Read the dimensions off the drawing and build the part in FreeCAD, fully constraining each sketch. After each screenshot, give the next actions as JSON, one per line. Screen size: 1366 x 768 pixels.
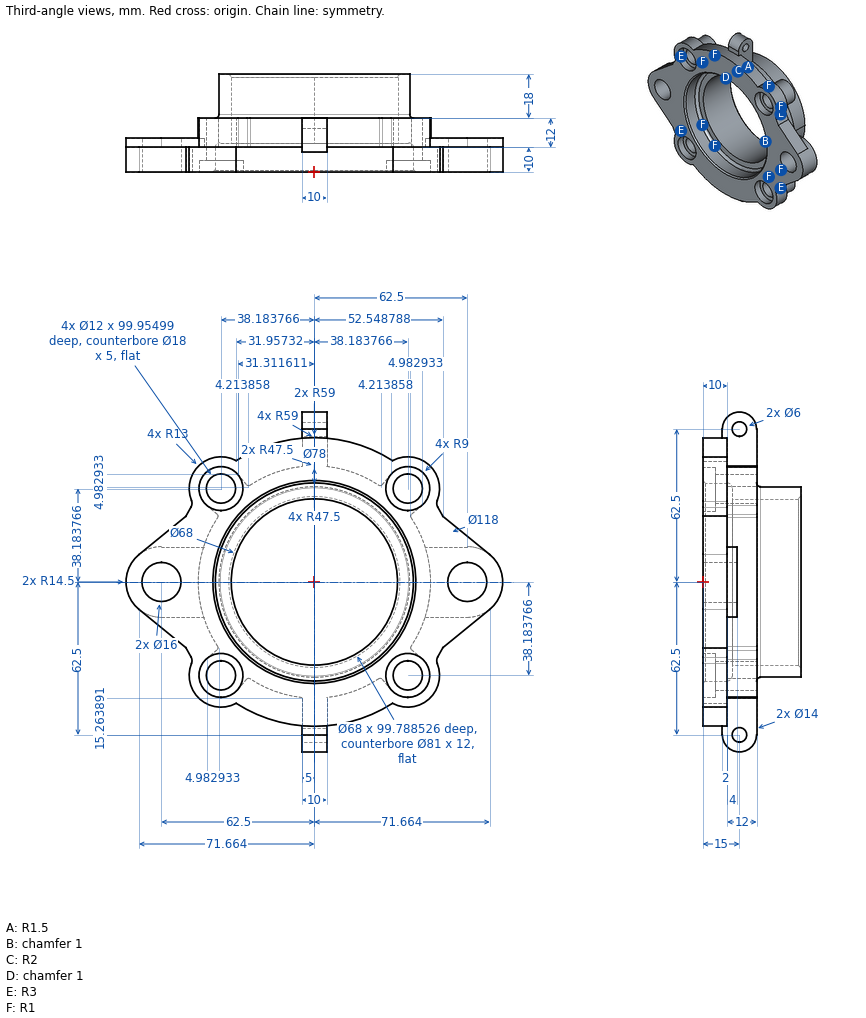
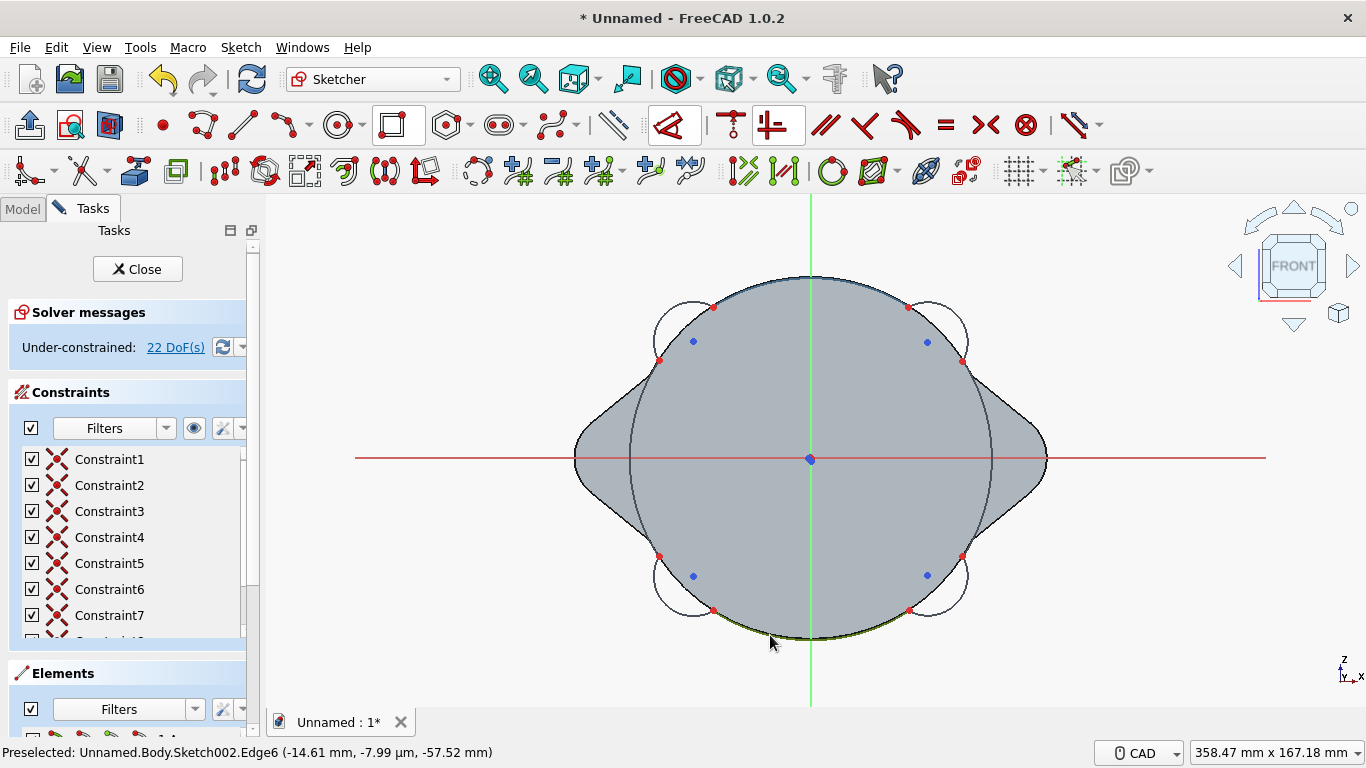
{"action": "left_click", "coordinate": [732, 126]}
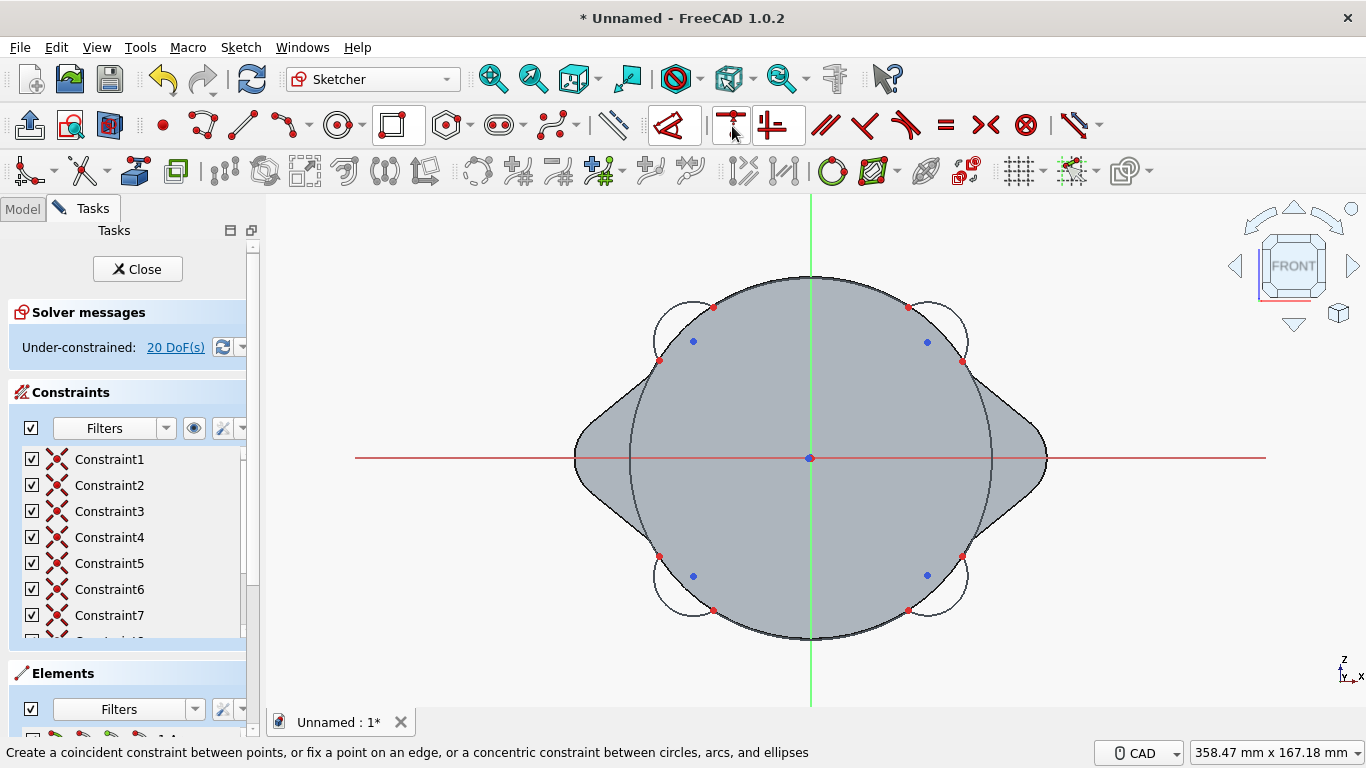
{"action": "left_click", "coordinate": [852, 283]}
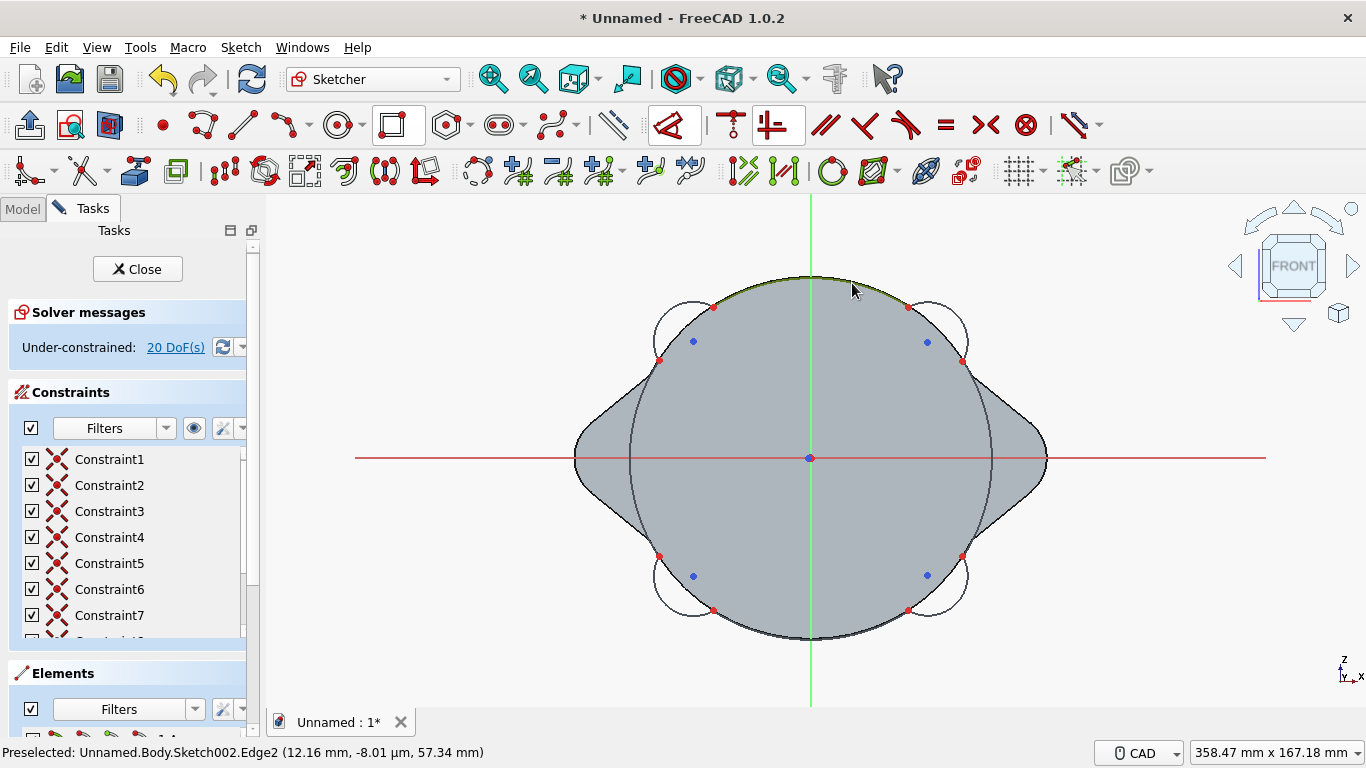
{"action": "left_click", "coordinate": [635, 418]}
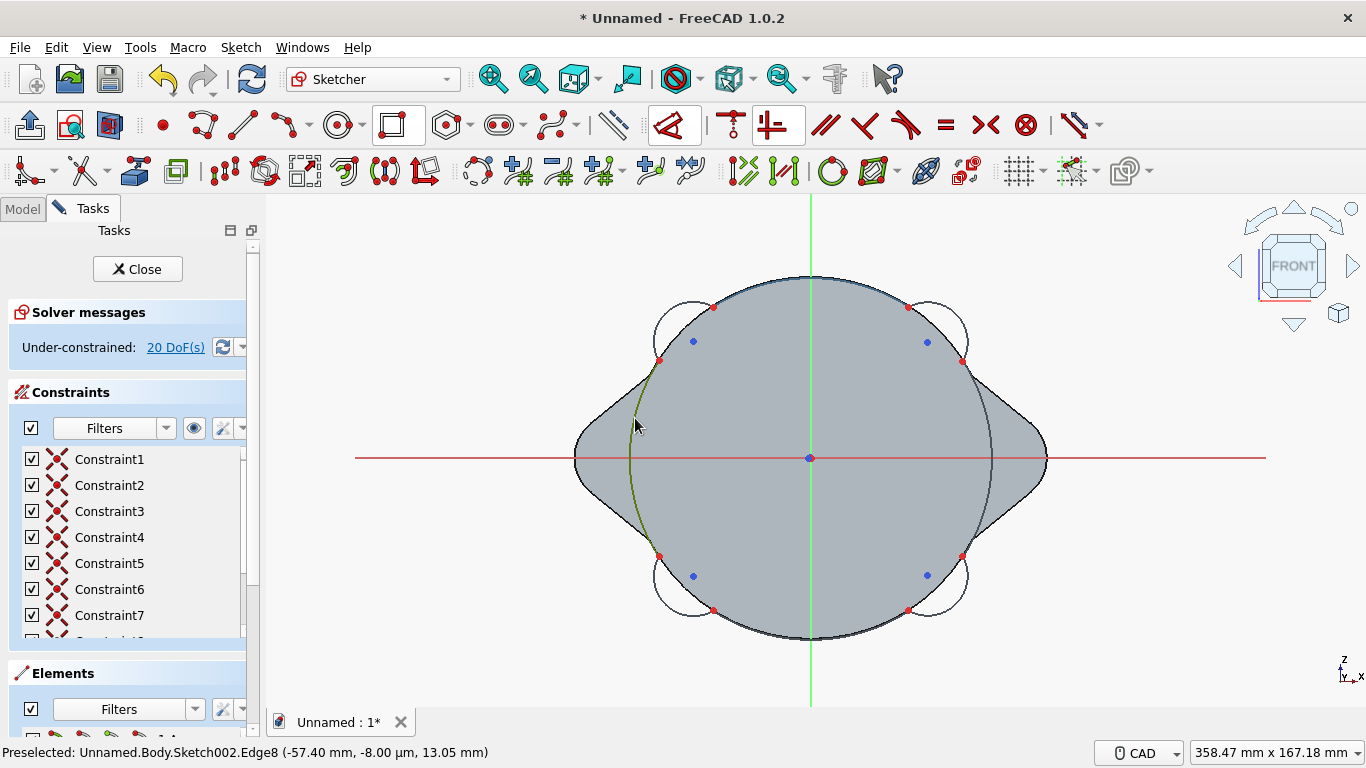
{"action": "left_click", "coordinate": [732, 126]}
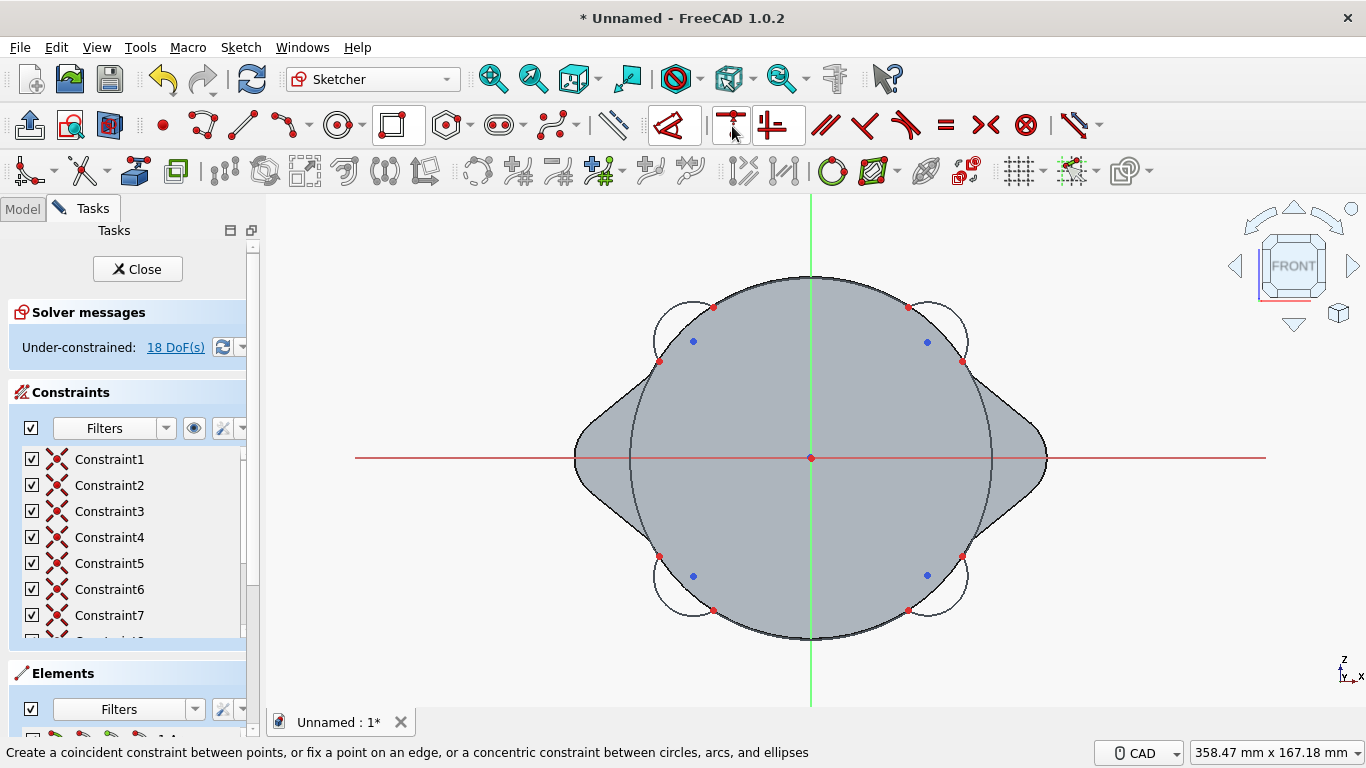
{"action": "left_click_drag", "start_coordinate": [801, 448], "coordinate": [821, 469]}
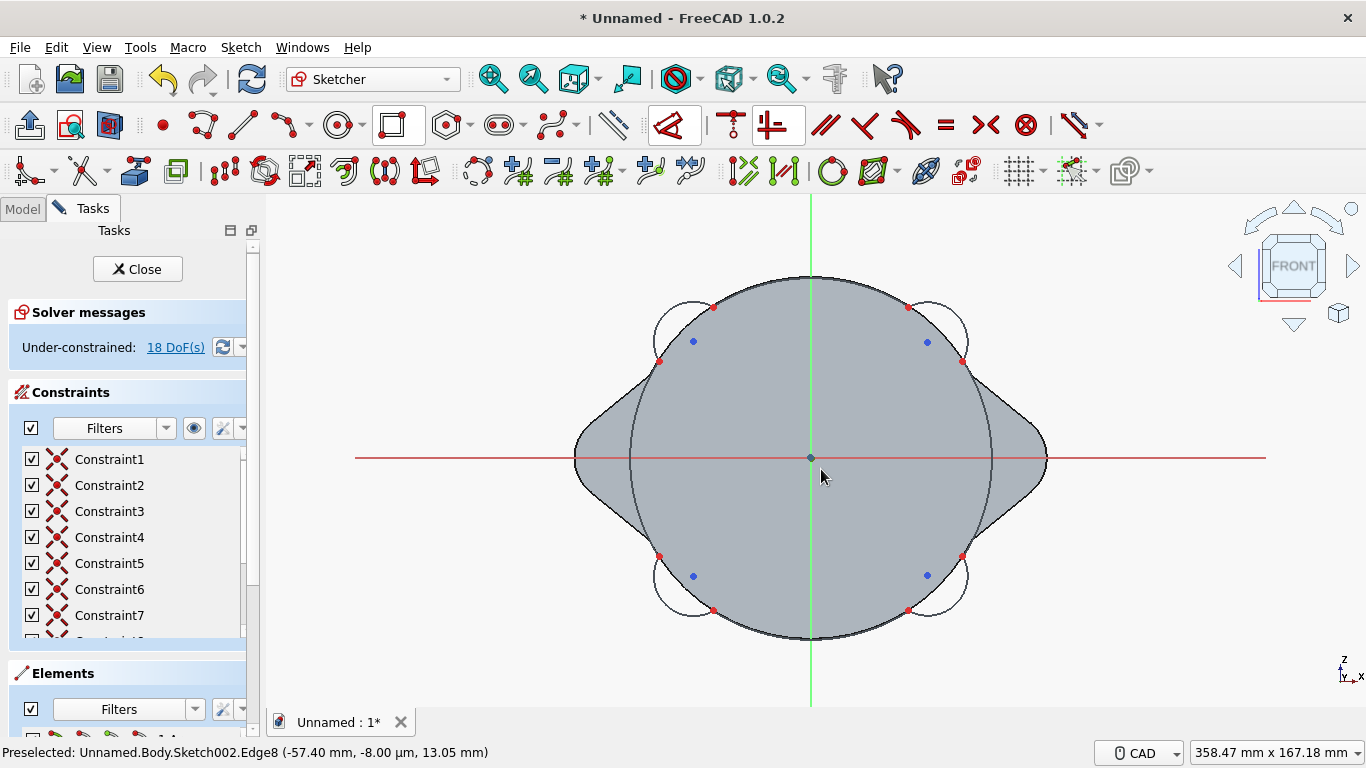
{"action": "left_click", "coordinate": [732, 126]}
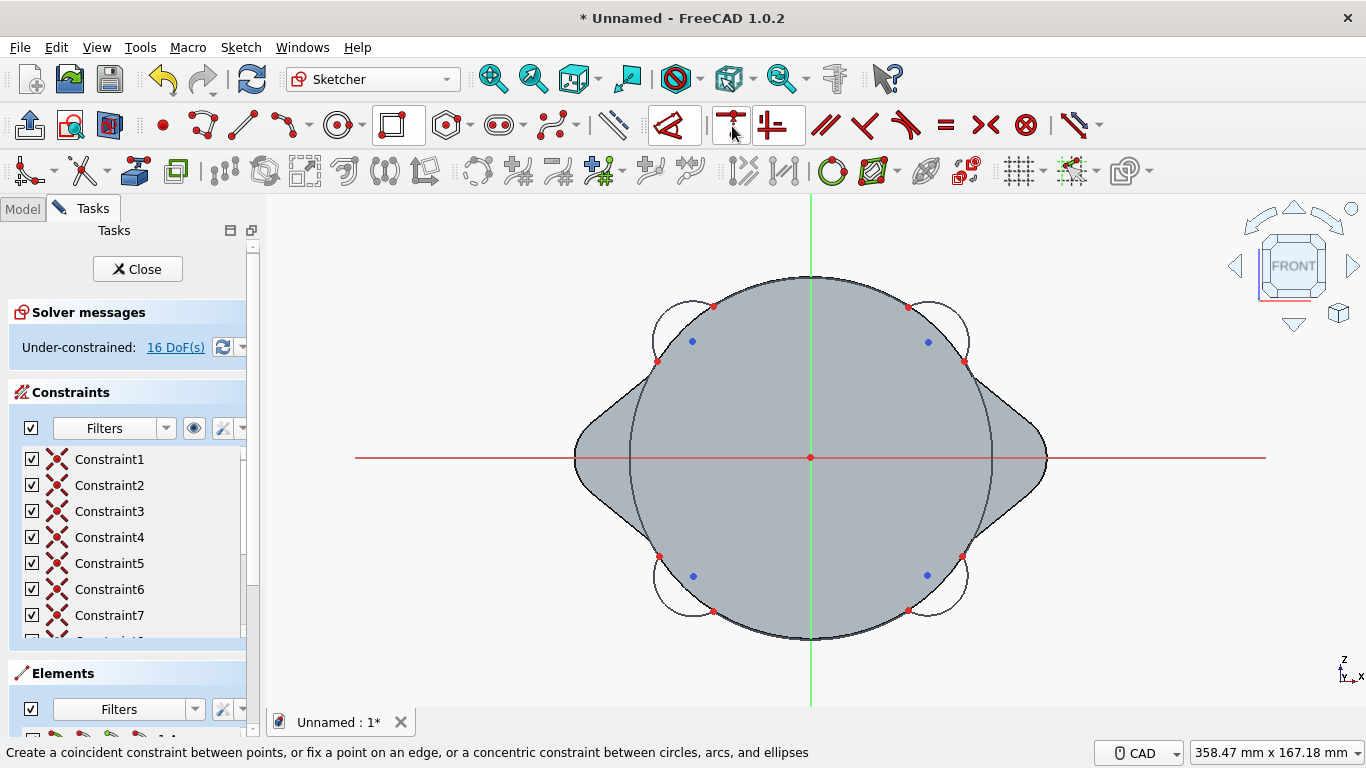
{"action": "left_click", "coordinate": [683, 303]}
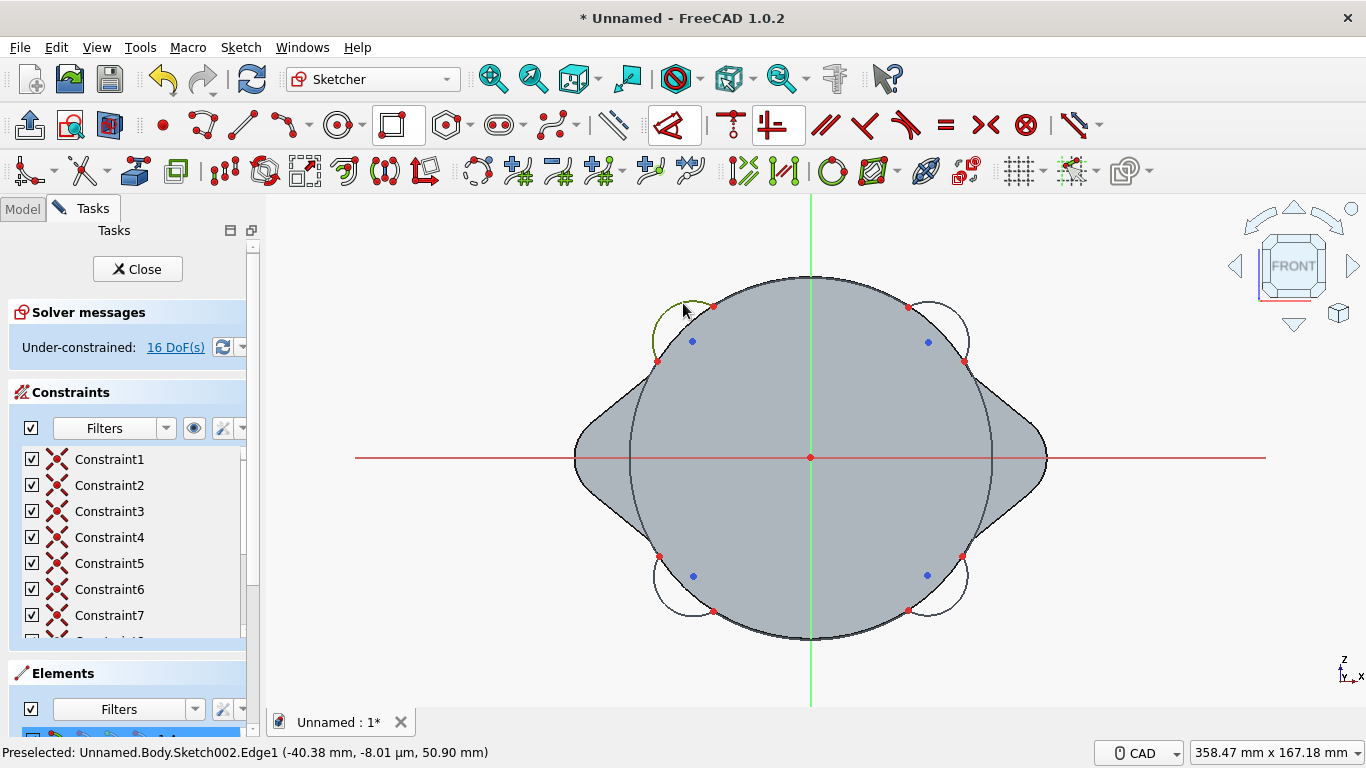
{"action": "left_click", "coordinate": [967, 331]}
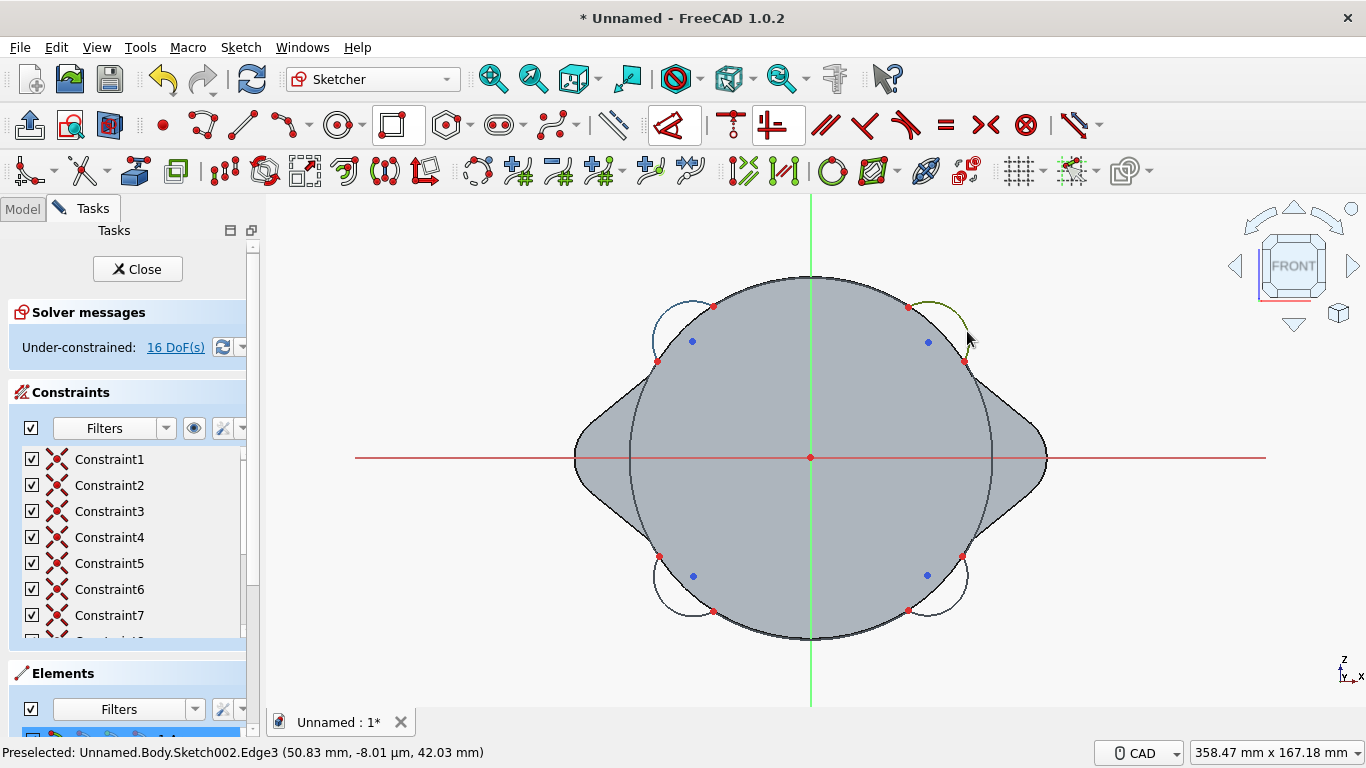
{"action": "left_click", "coordinate": [939, 614]}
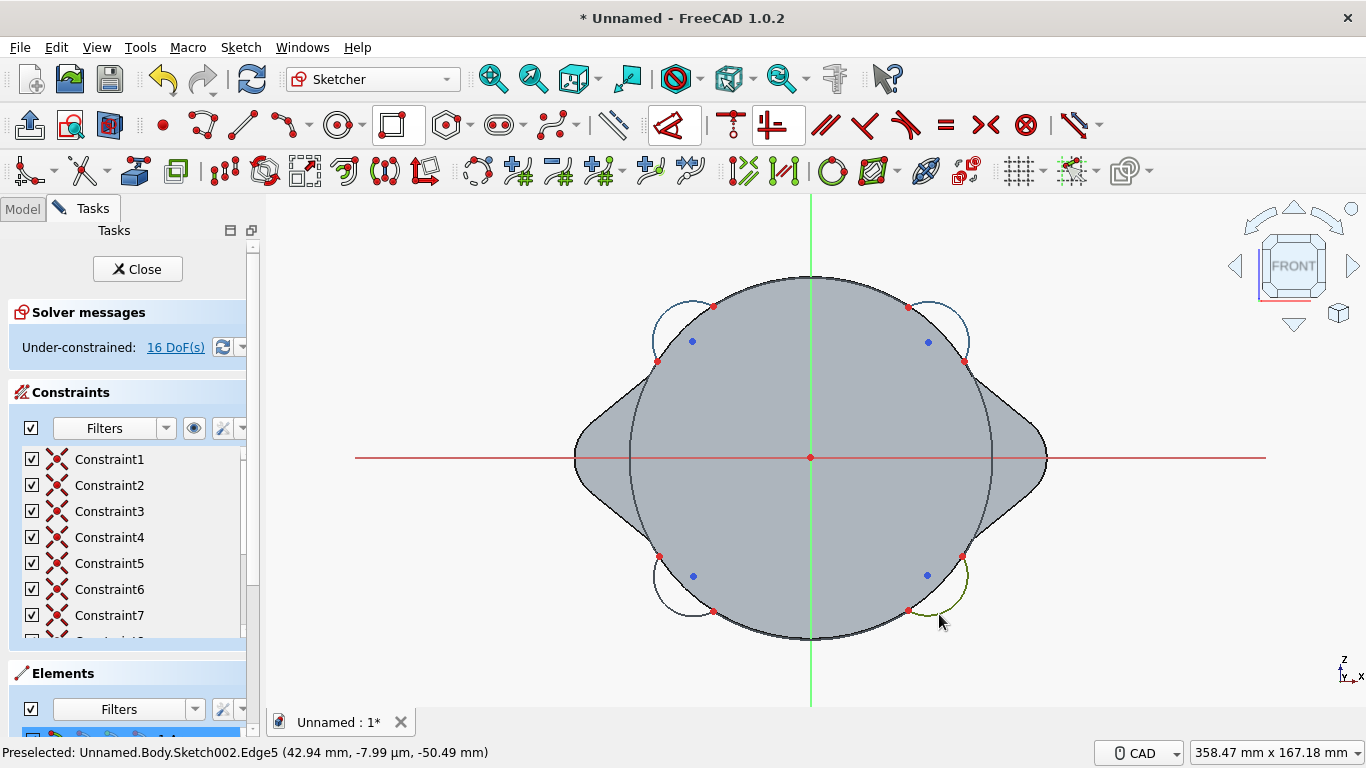
{"action": "left_click", "coordinate": [655, 587]}